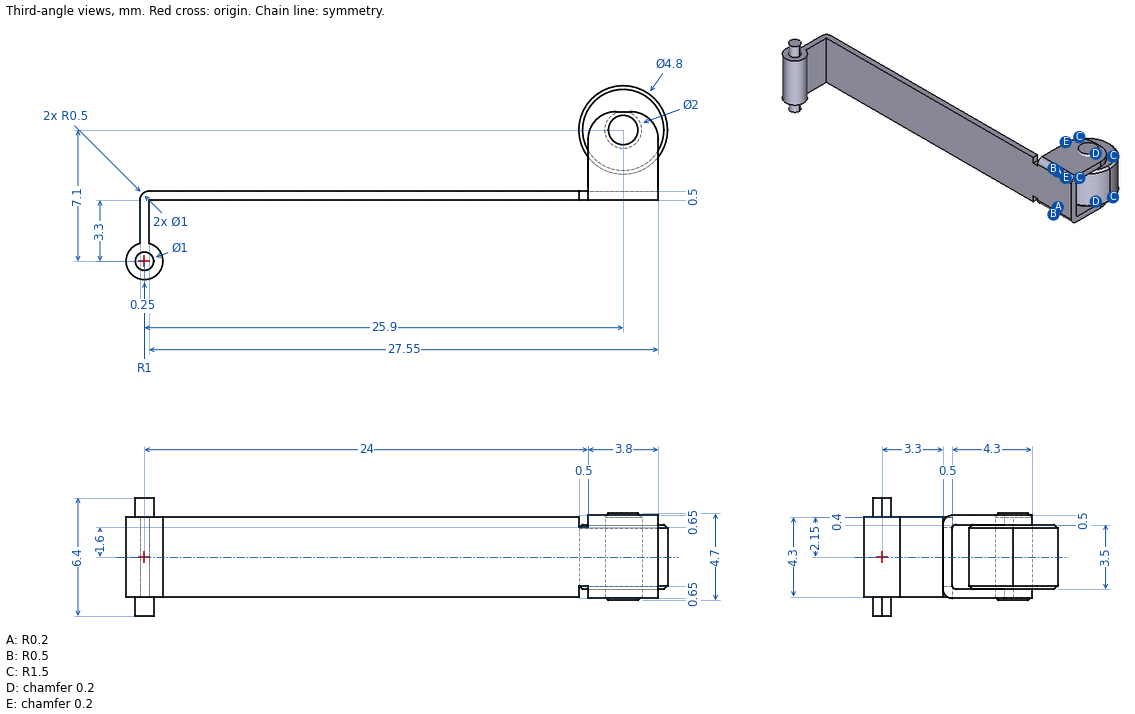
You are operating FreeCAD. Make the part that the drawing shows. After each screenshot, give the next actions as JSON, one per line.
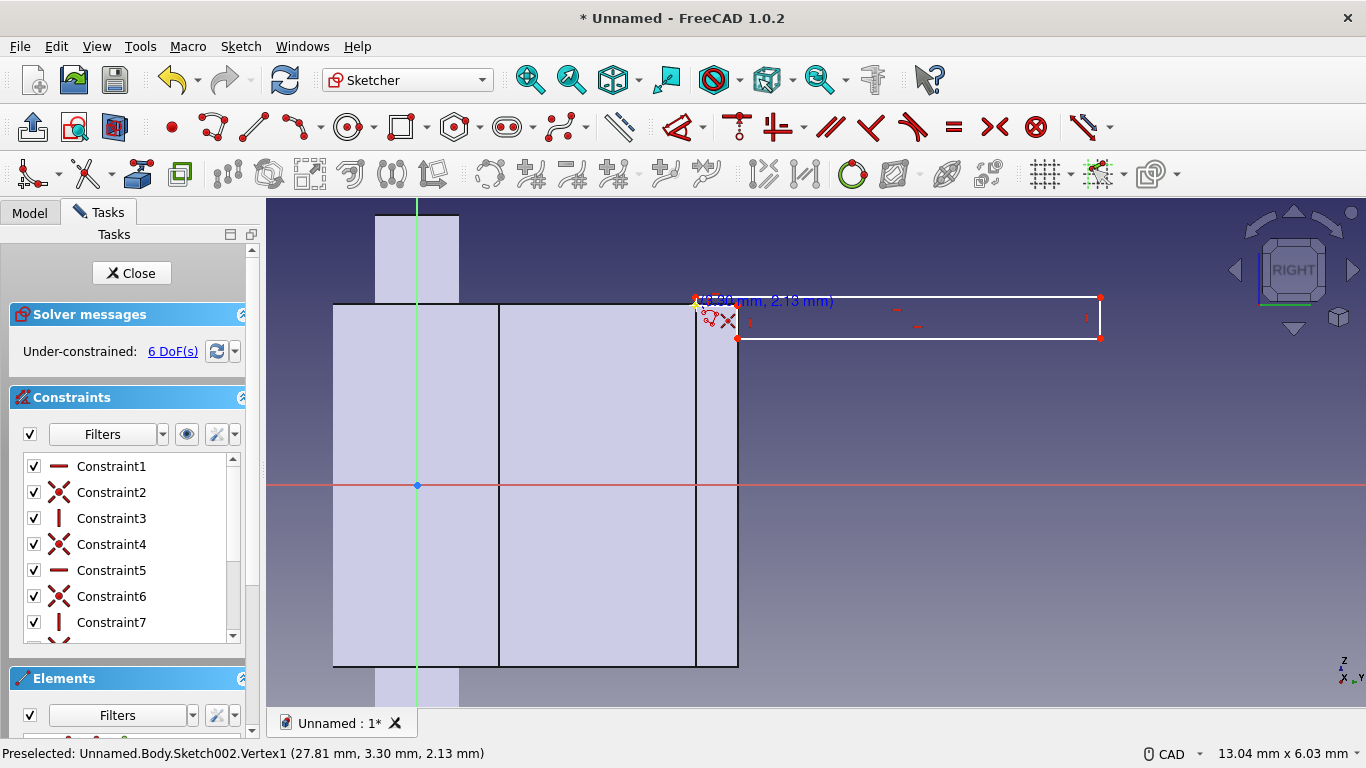
{"action": "left_click", "coordinate": [696, 601]}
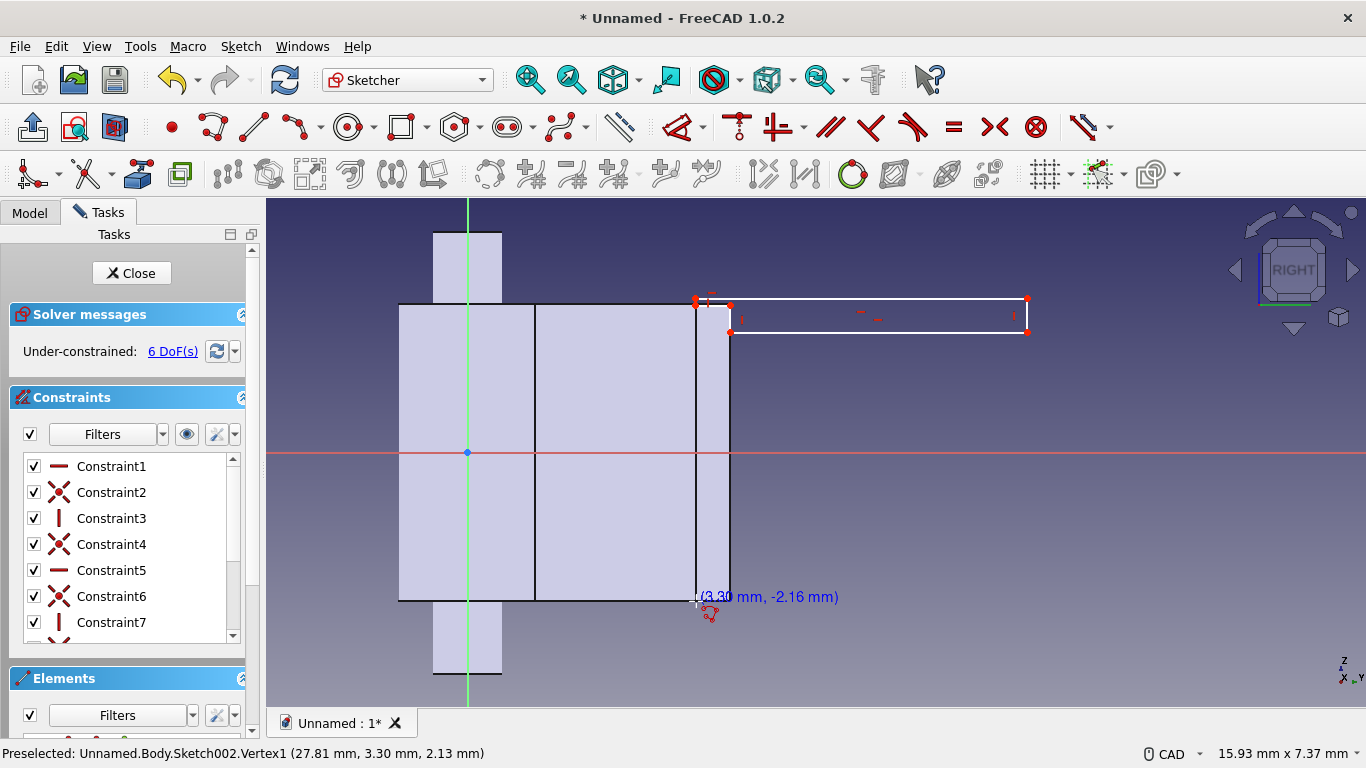
{"action": "scroll", "coordinate": [696, 608], "scroll_direction": "up", "scroll_amount": 5}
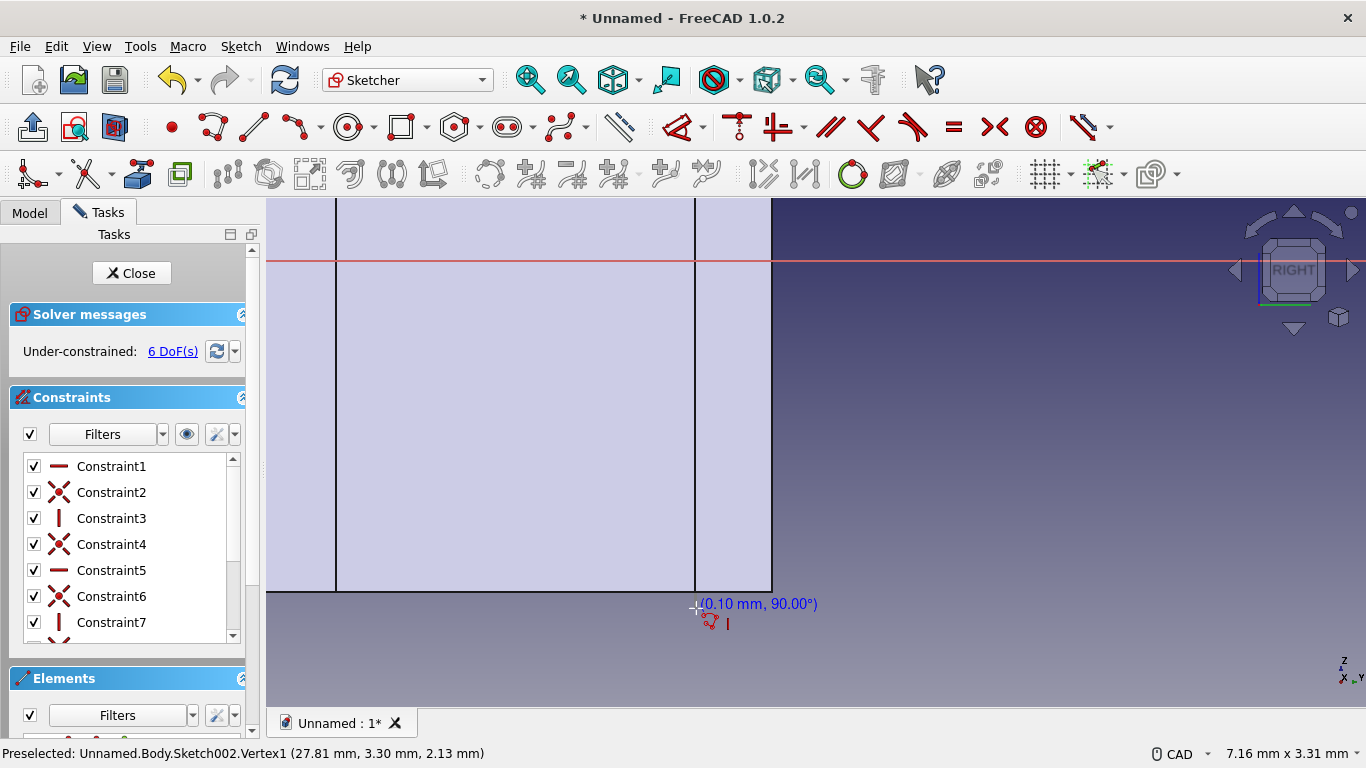
{"action": "left_click", "coordinate": [695, 607]}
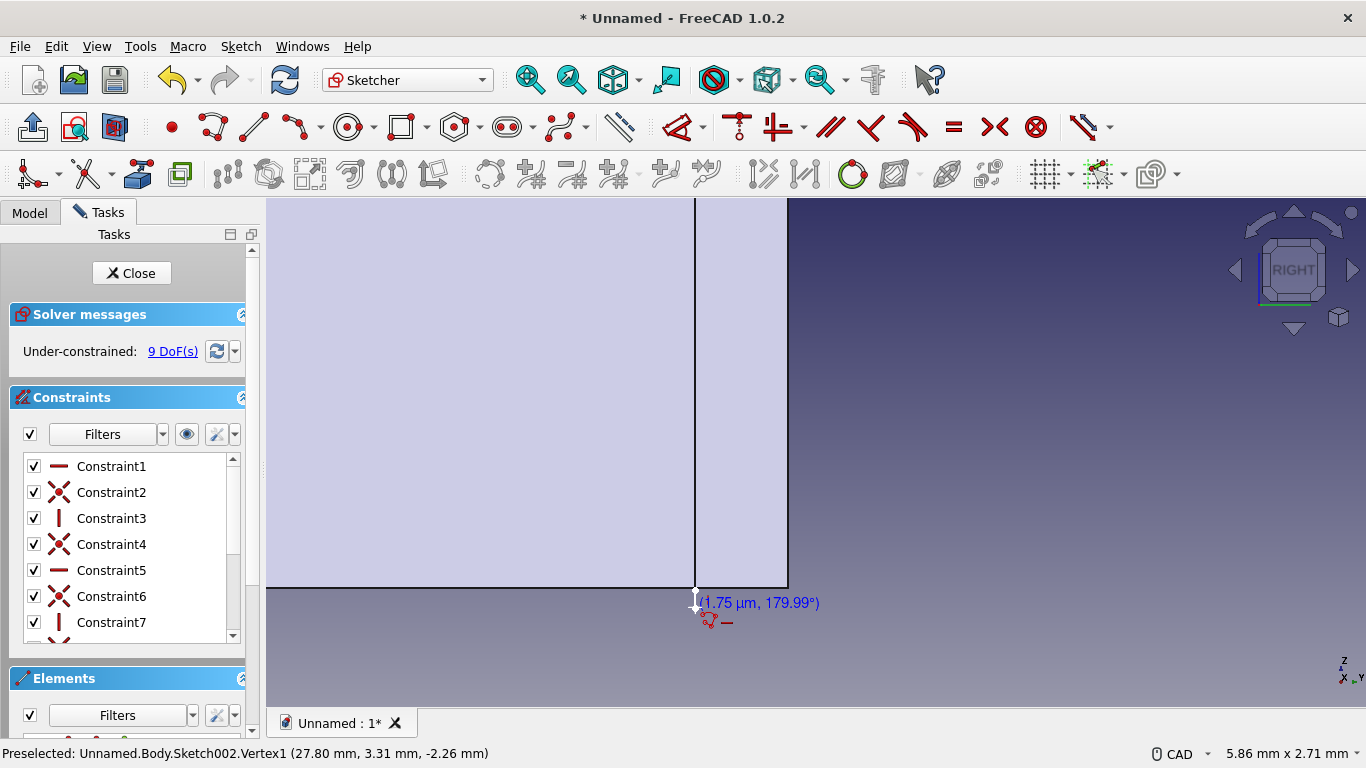
{"action": "scroll", "coordinate": [696, 608], "scroll_direction": "down", "scroll_amount": 5}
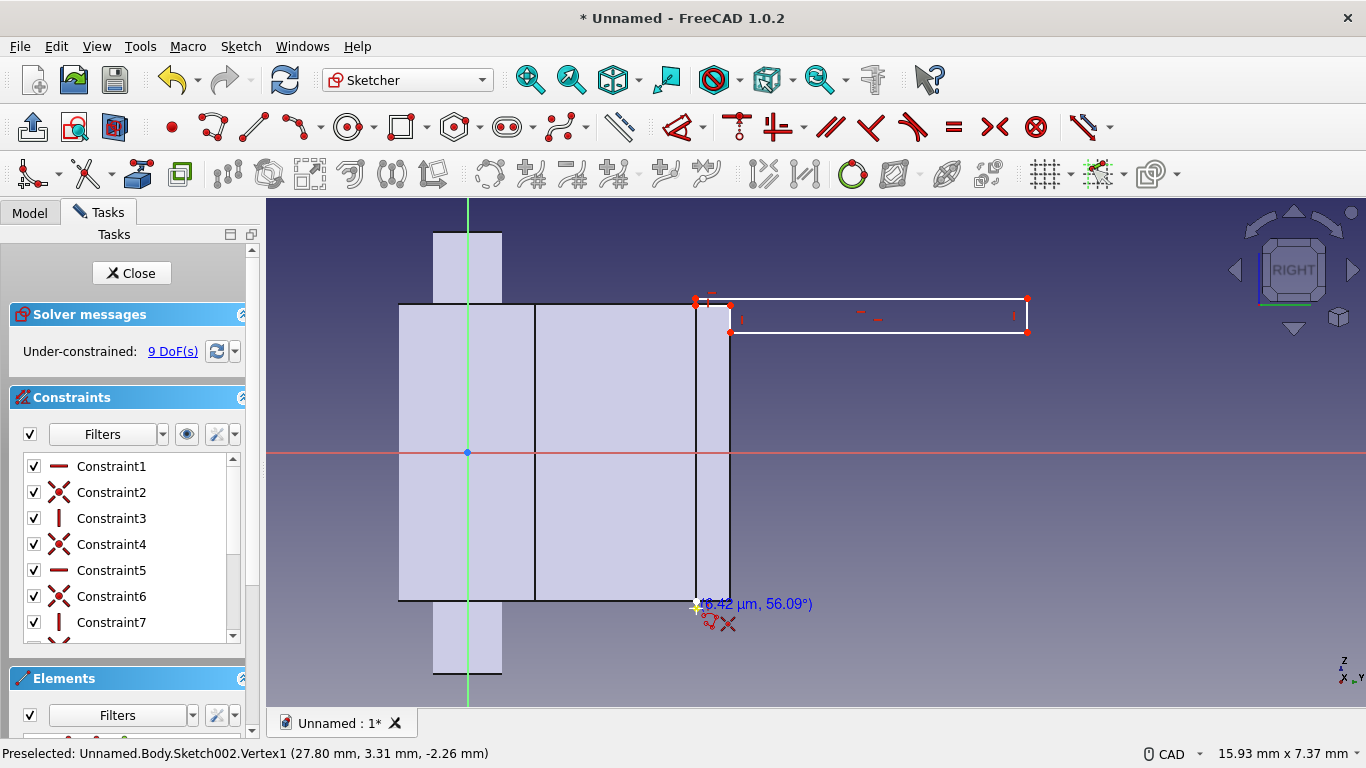
{"action": "left_click", "coordinate": [1027, 608]}
{"action": "left_click", "coordinate": [1027, 574]}
{"action": "left_click", "coordinate": [730, 574]}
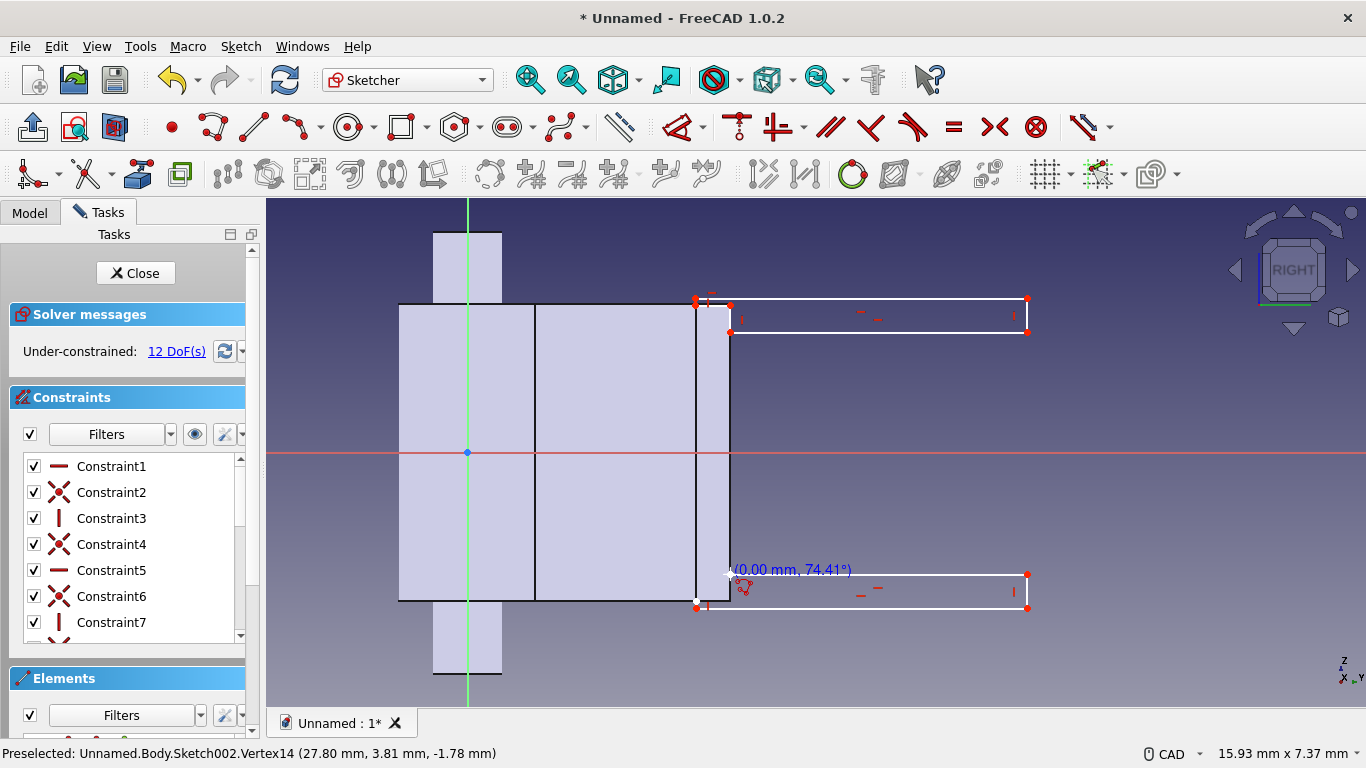
{"action": "scroll", "coordinate": [730, 601], "scroll_direction": "up", "scroll_amount": 5}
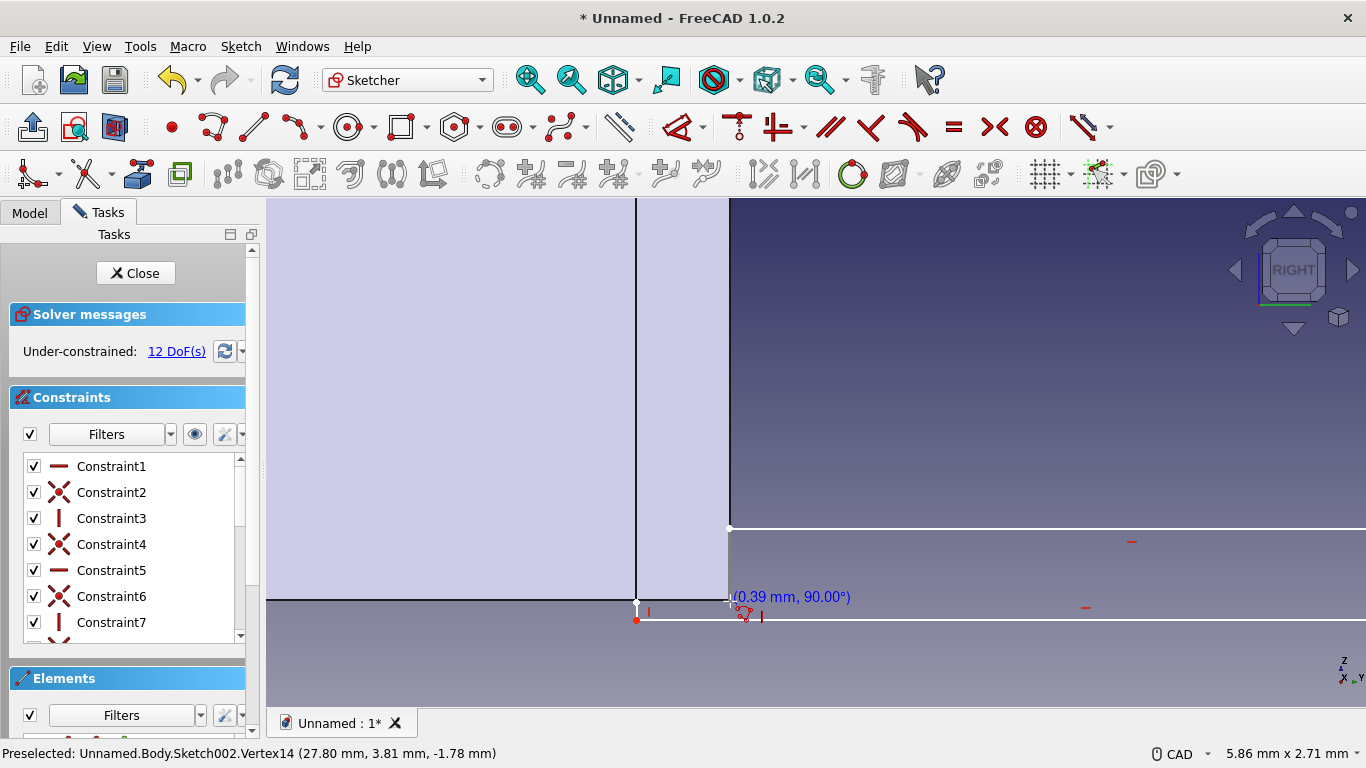
{"action": "left_click", "coordinate": [729, 600]}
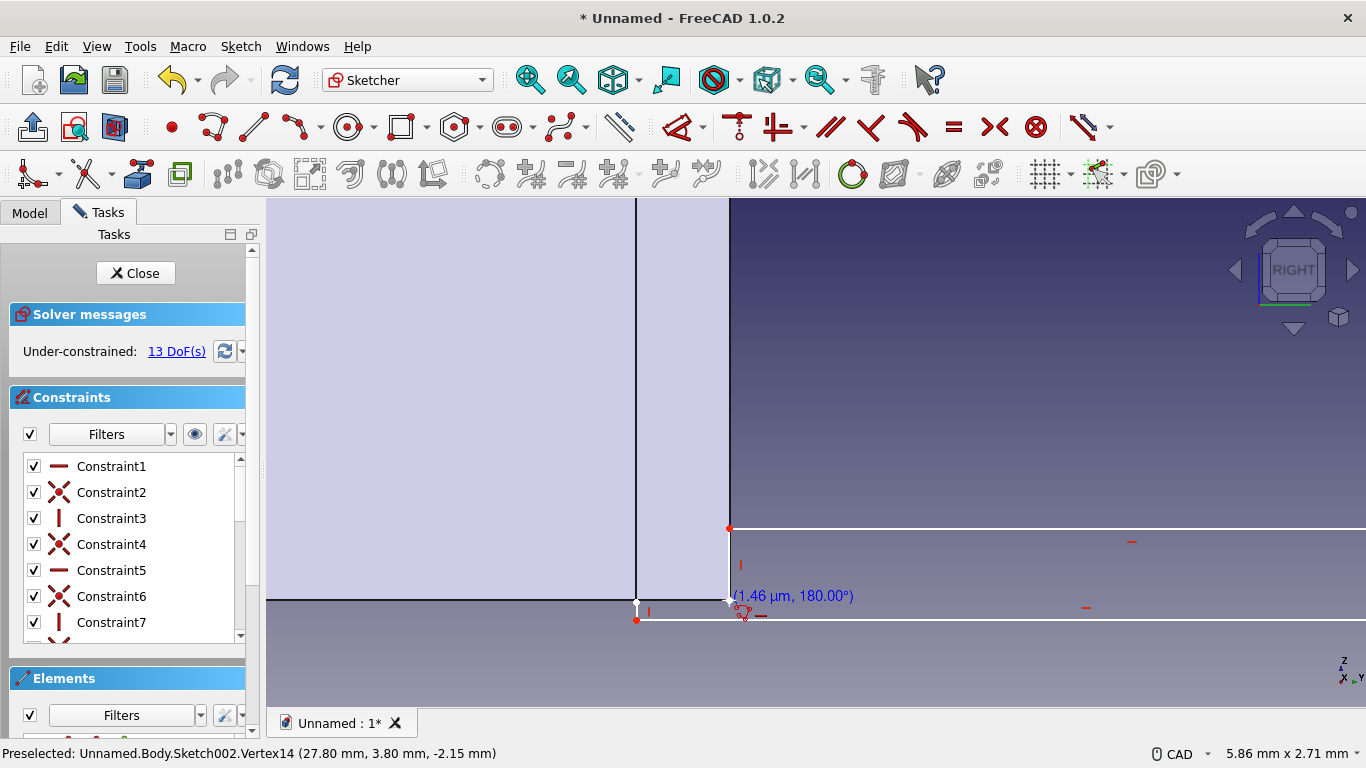
{"action": "scroll", "coordinate": [636, 600], "scroll_direction": "up", "scroll_amount": 3}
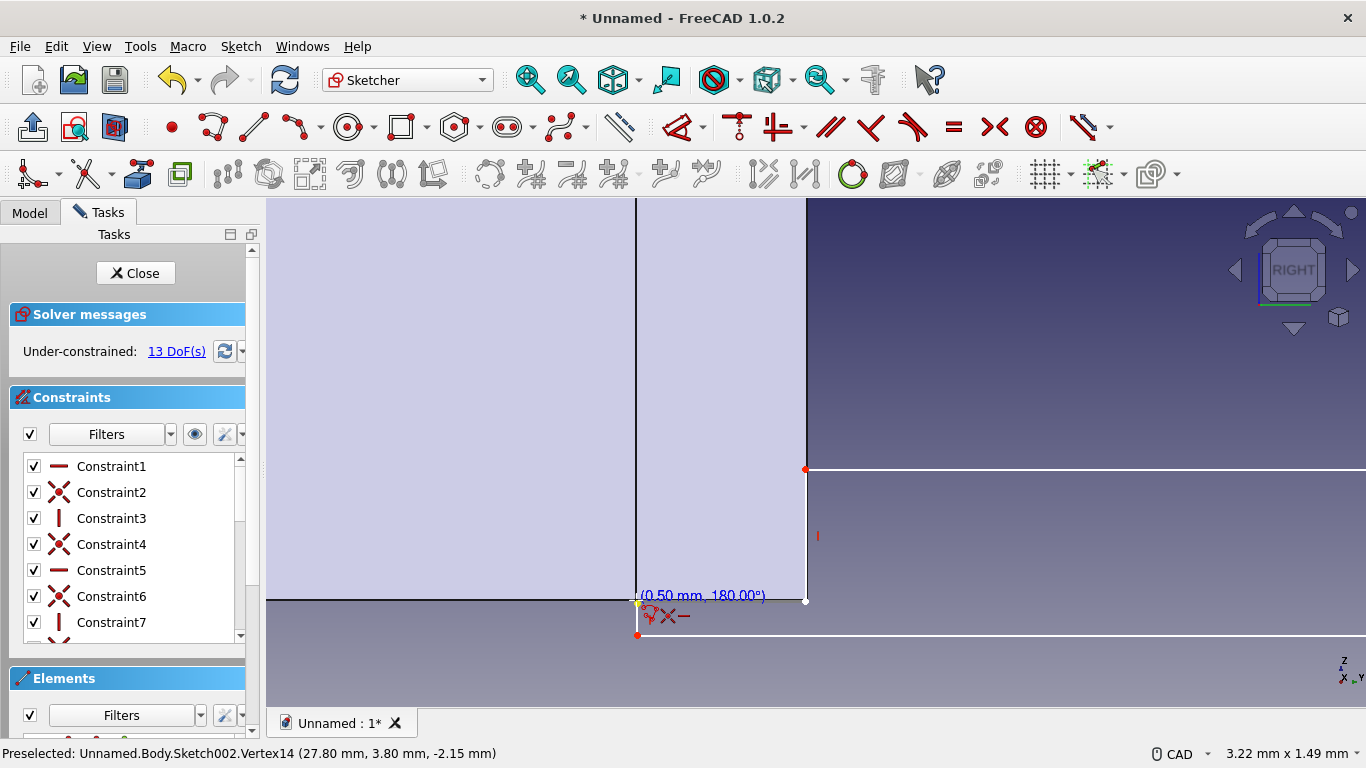
{"action": "left_click", "coordinate": [637, 604]}
{"action": "key", "text": "Escape"}
{"action": "key", "text": "Escape"}